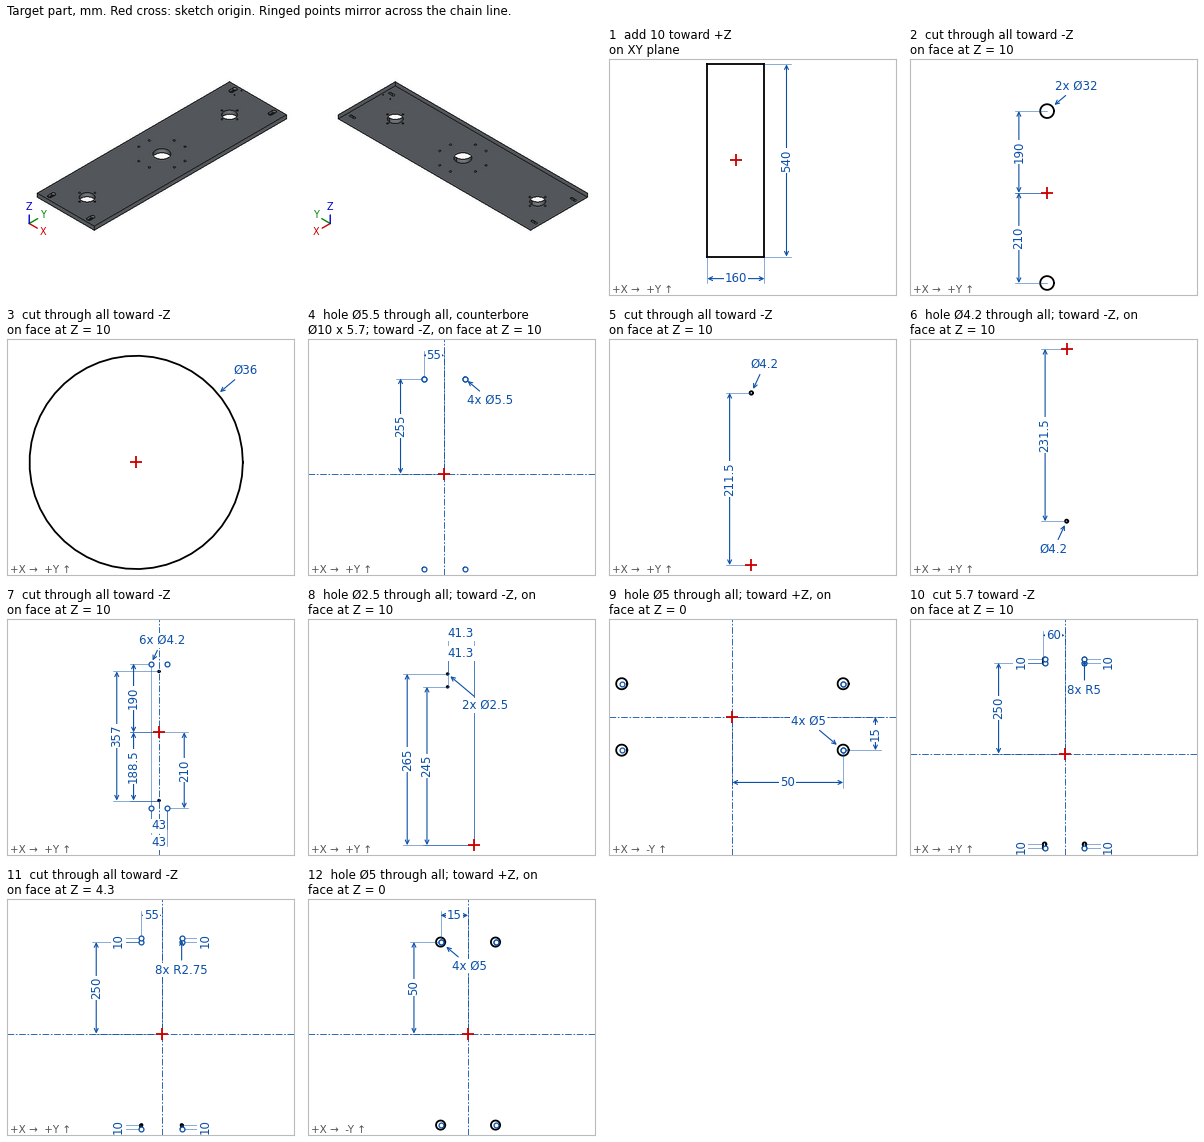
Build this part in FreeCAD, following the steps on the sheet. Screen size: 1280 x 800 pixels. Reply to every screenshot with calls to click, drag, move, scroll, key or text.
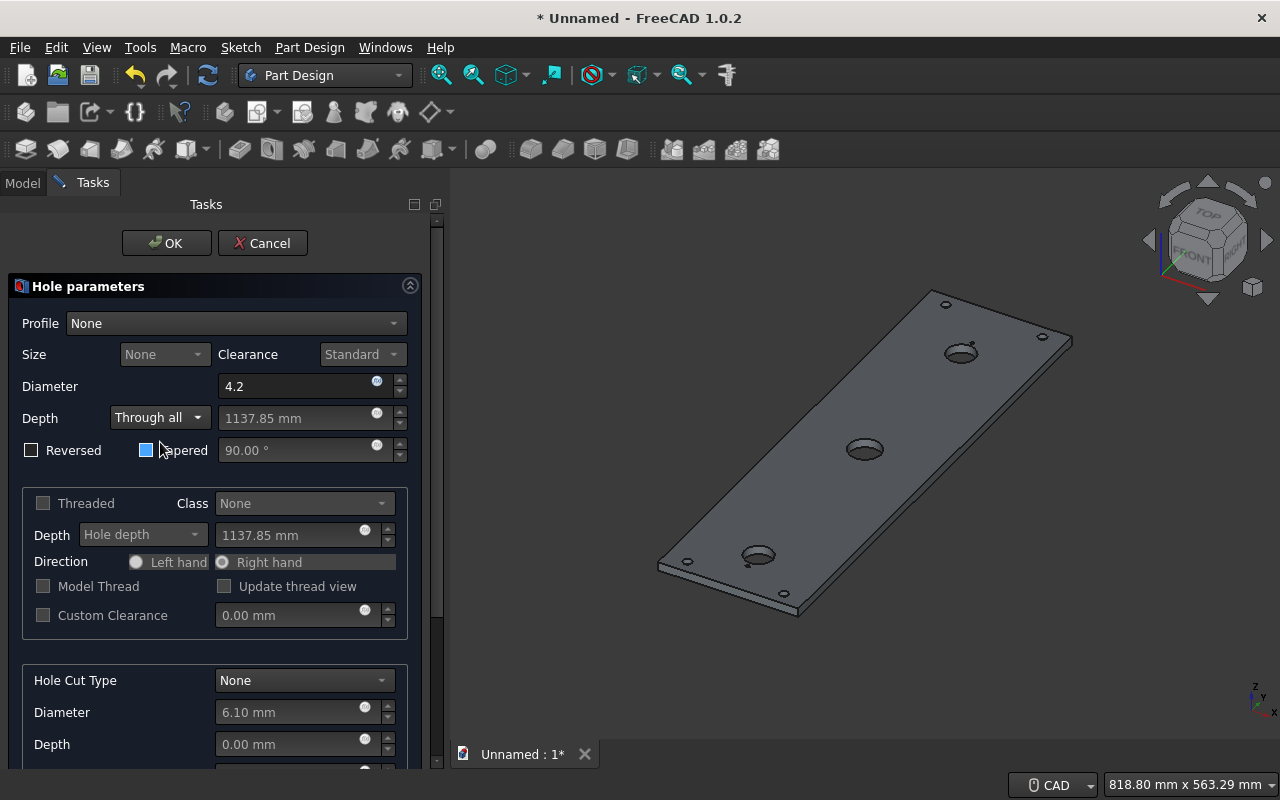
click(167, 243)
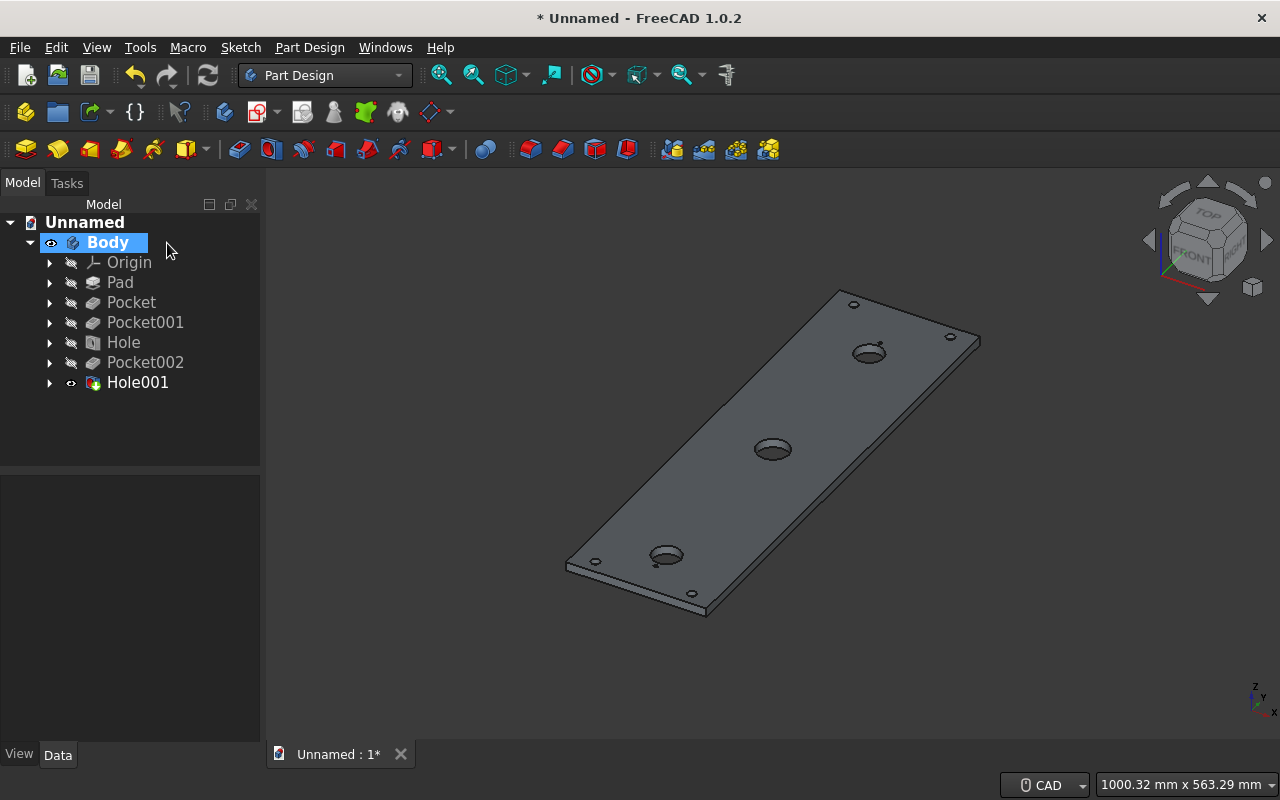
click(812, 410)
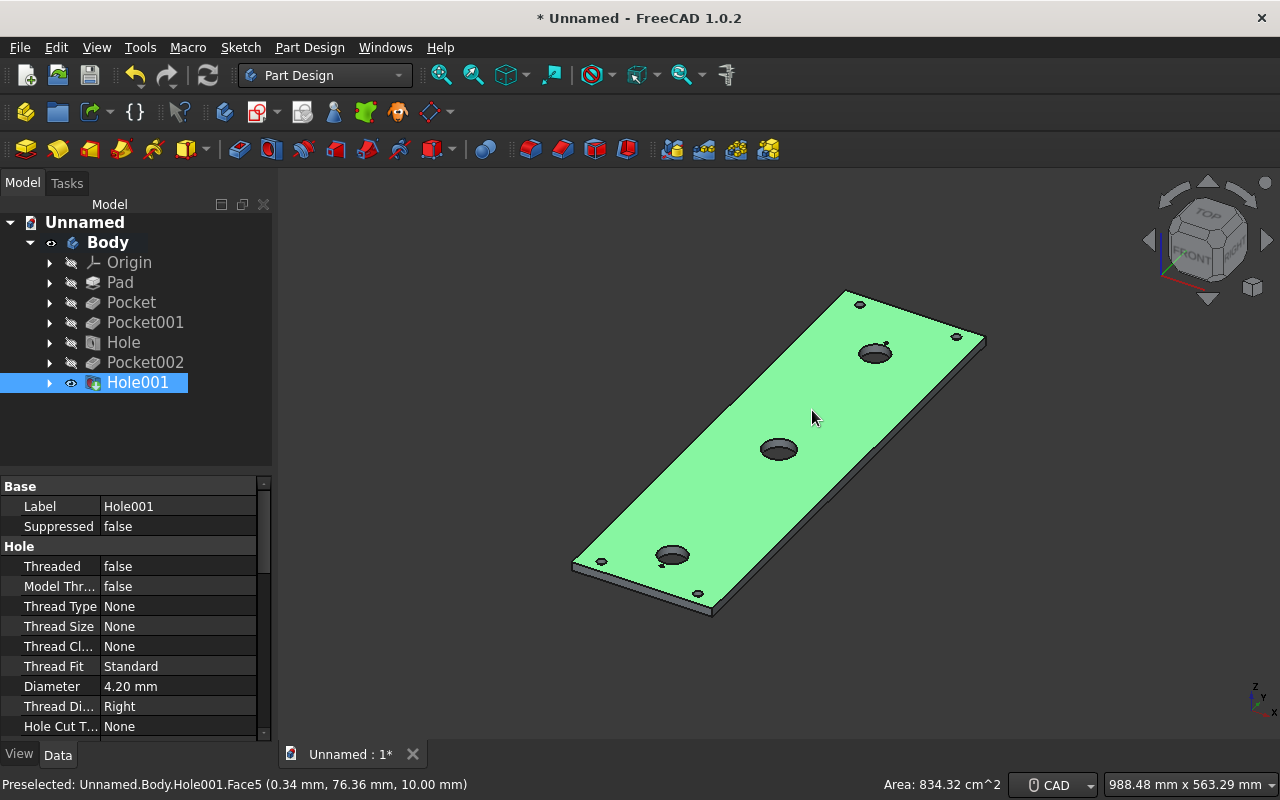
click(258, 112)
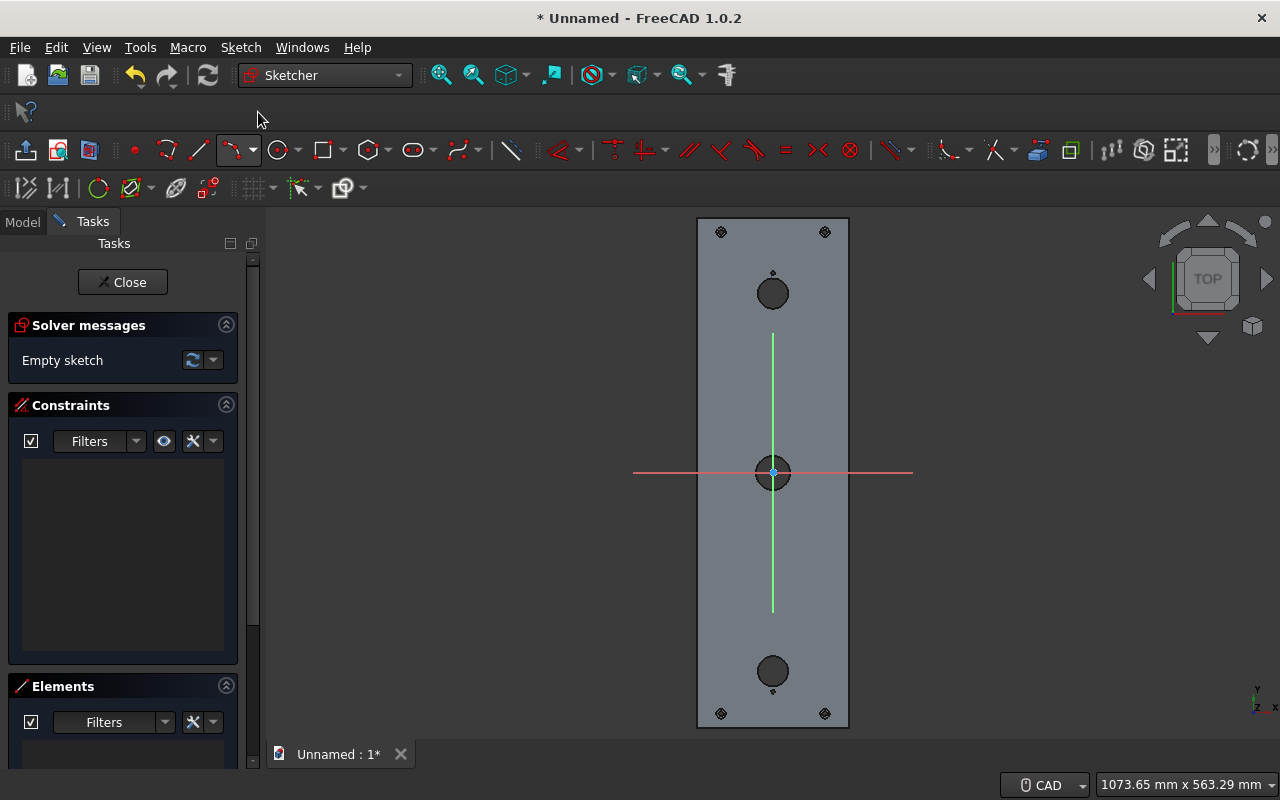
key(g)
key(c)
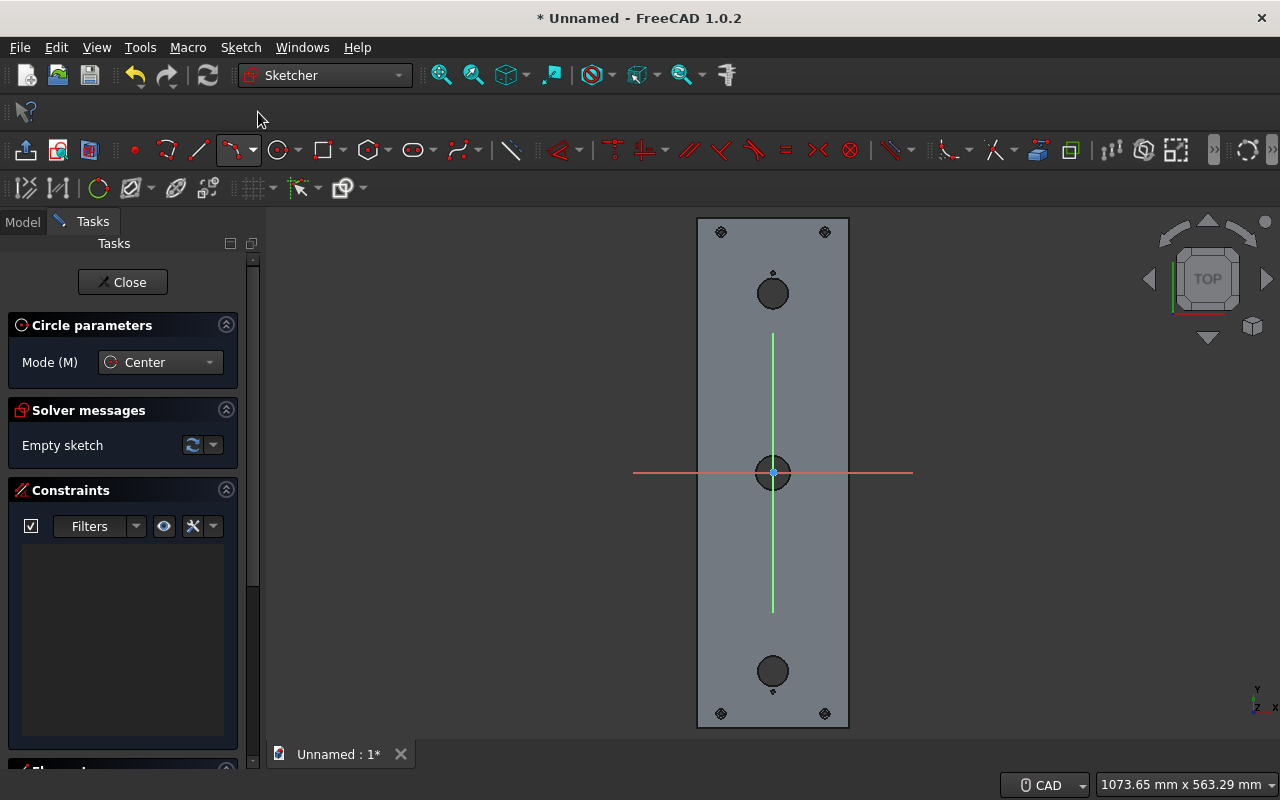
scroll(793, 671, up, 13)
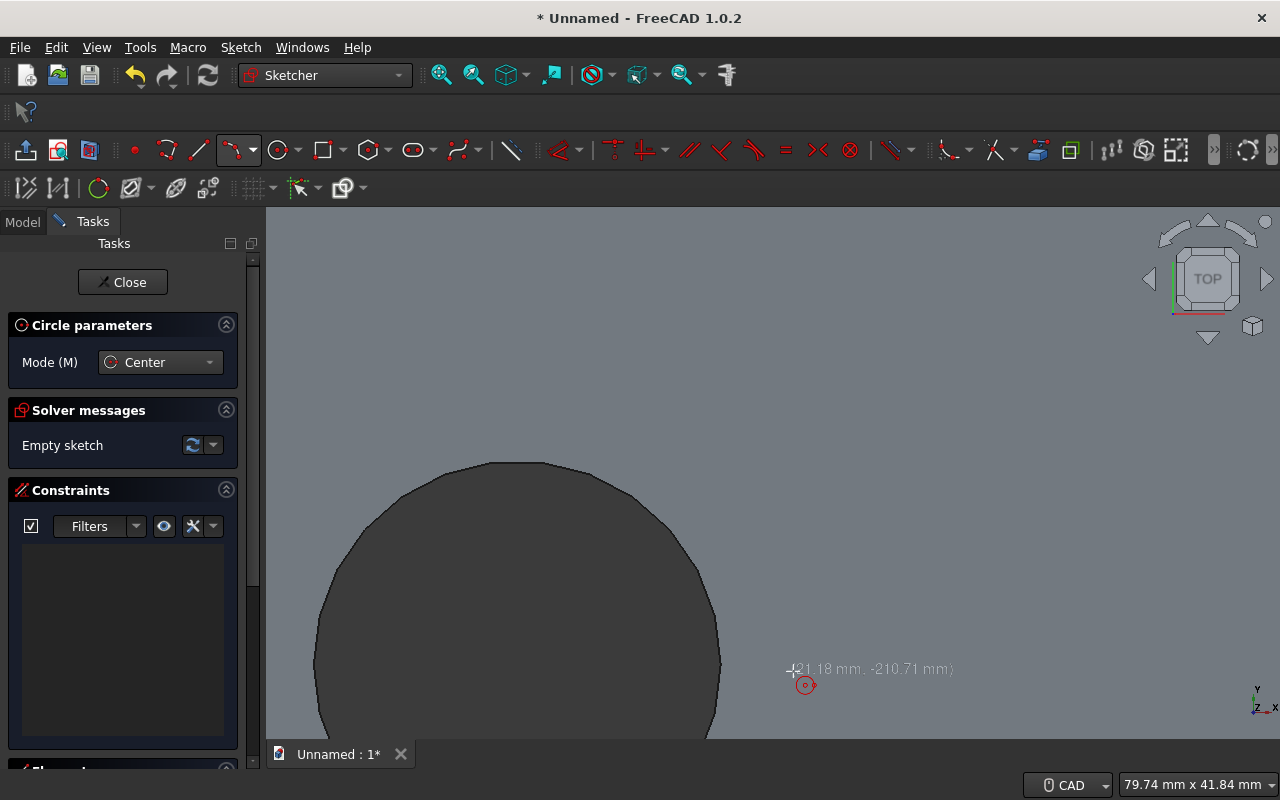
scroll(717, 625, down, 14)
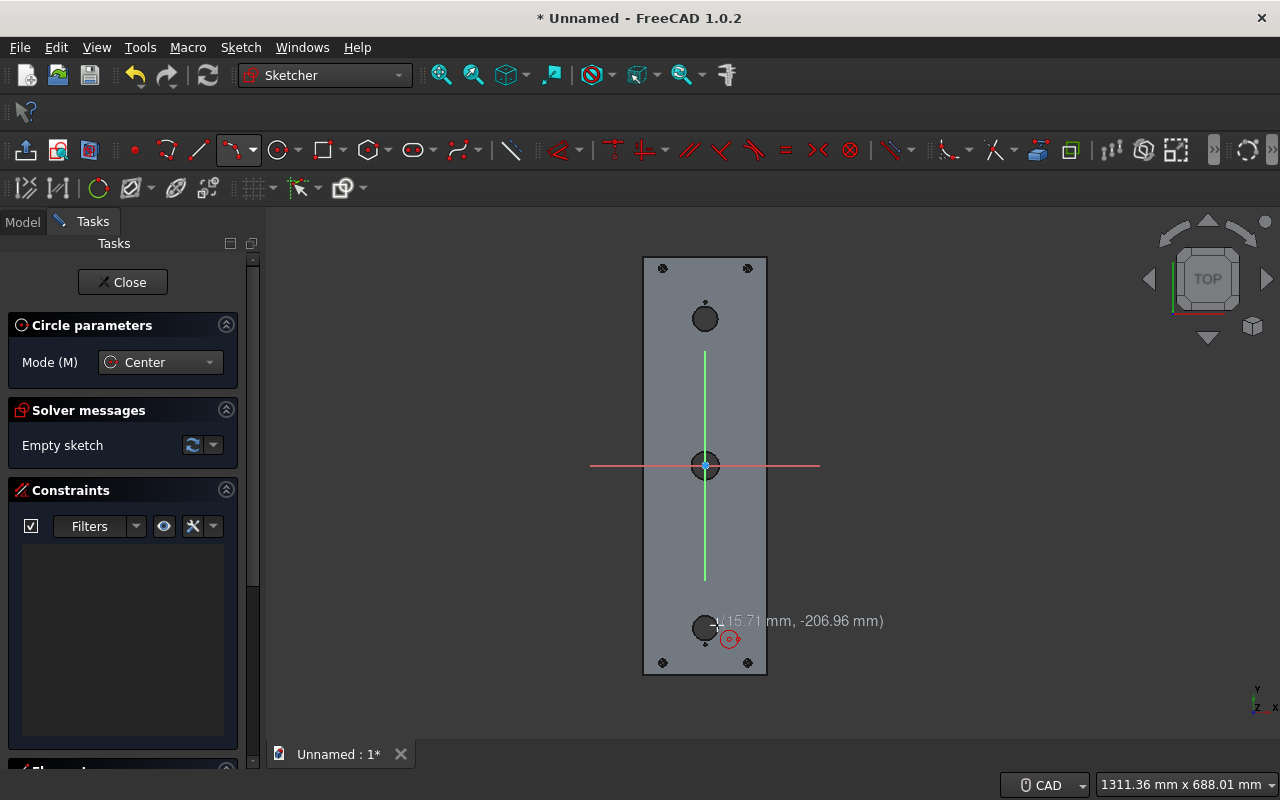
click(722, 628)
move(723, 627)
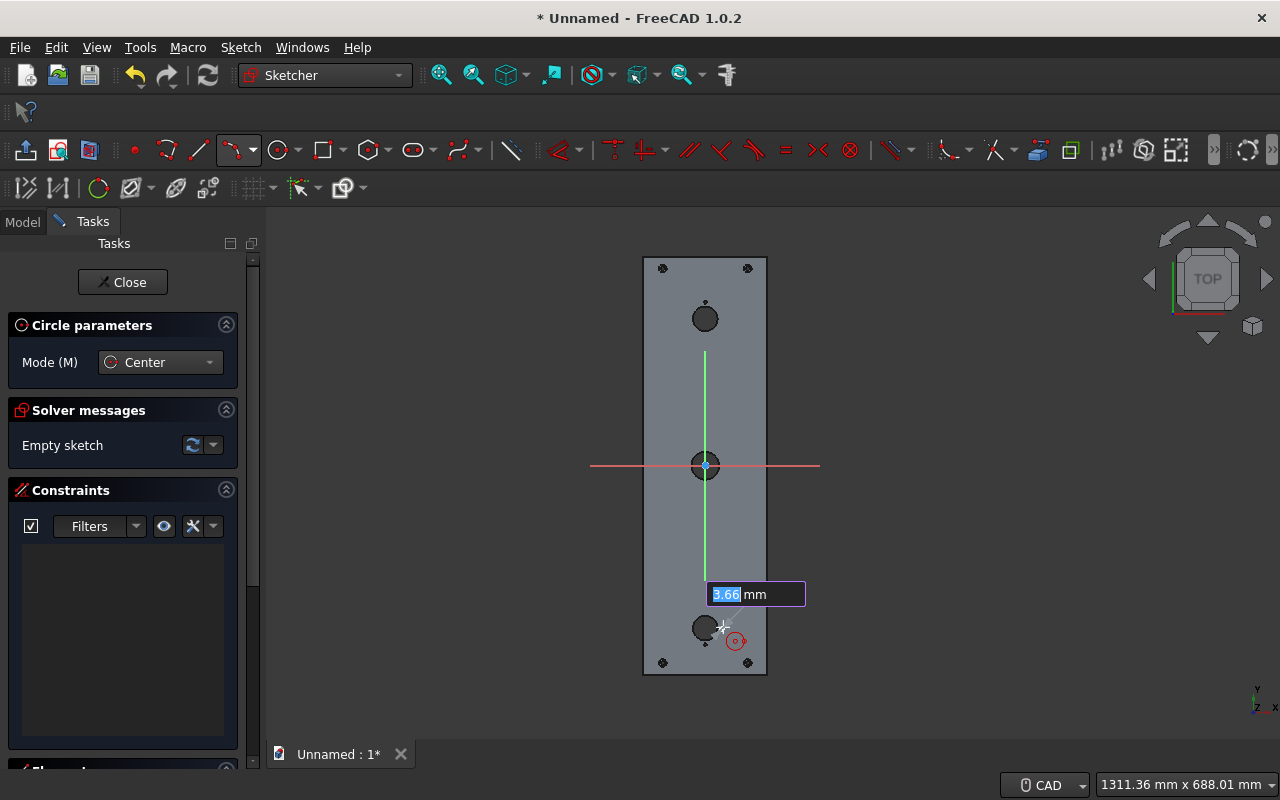
text(4.2)
key(Return)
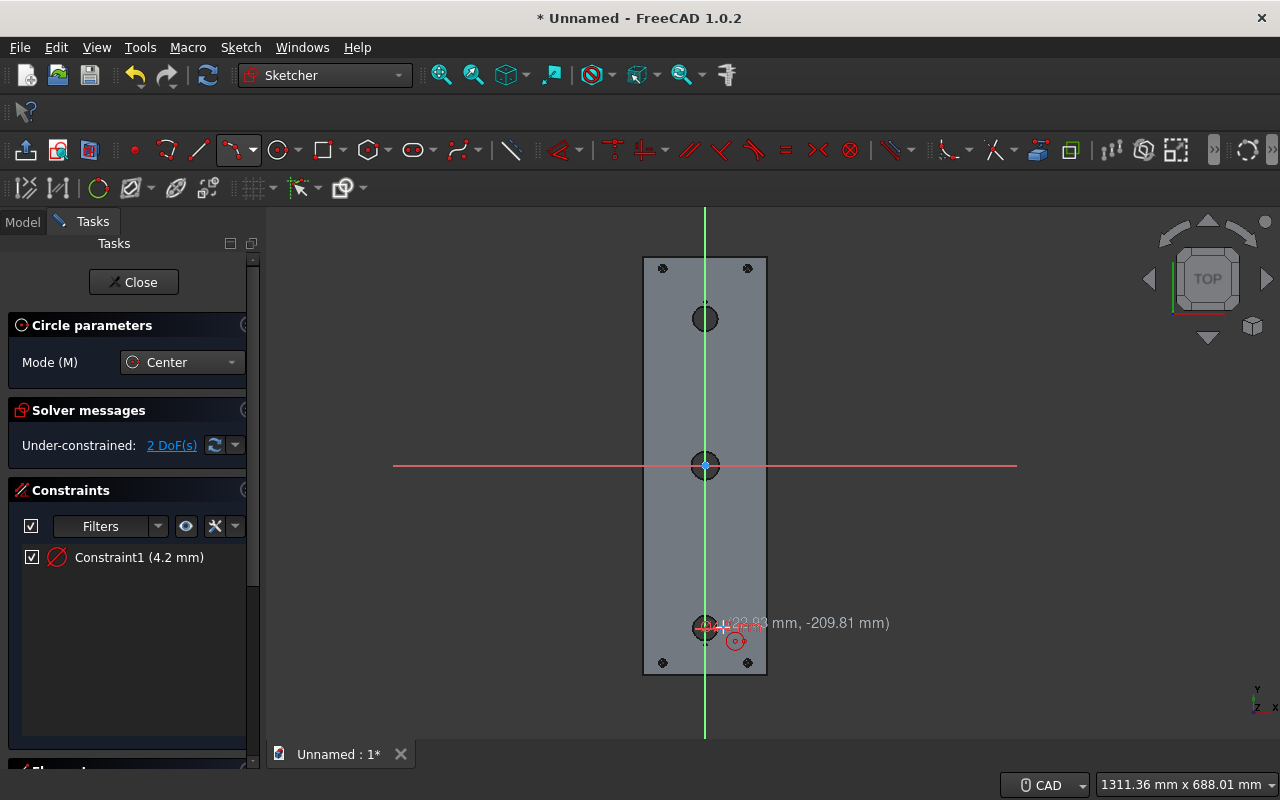
scroll(689, 628, up, 14)